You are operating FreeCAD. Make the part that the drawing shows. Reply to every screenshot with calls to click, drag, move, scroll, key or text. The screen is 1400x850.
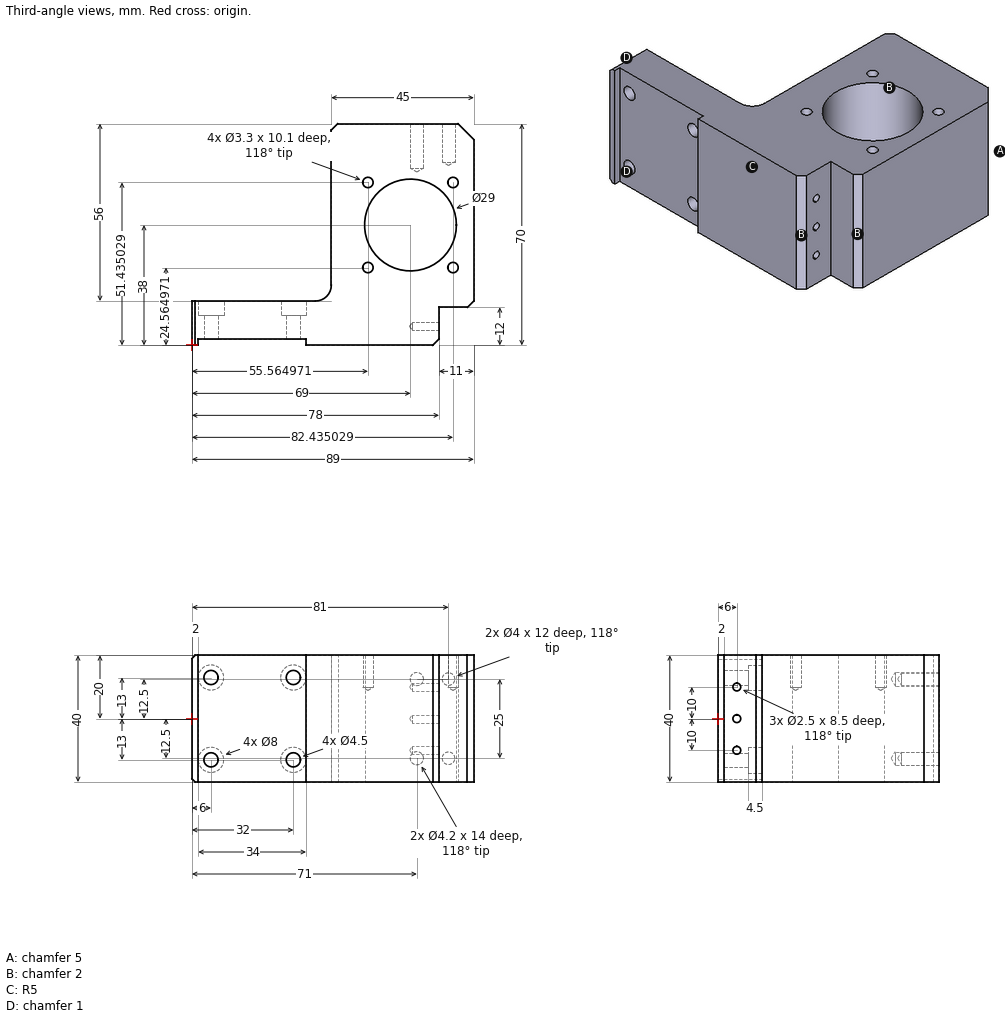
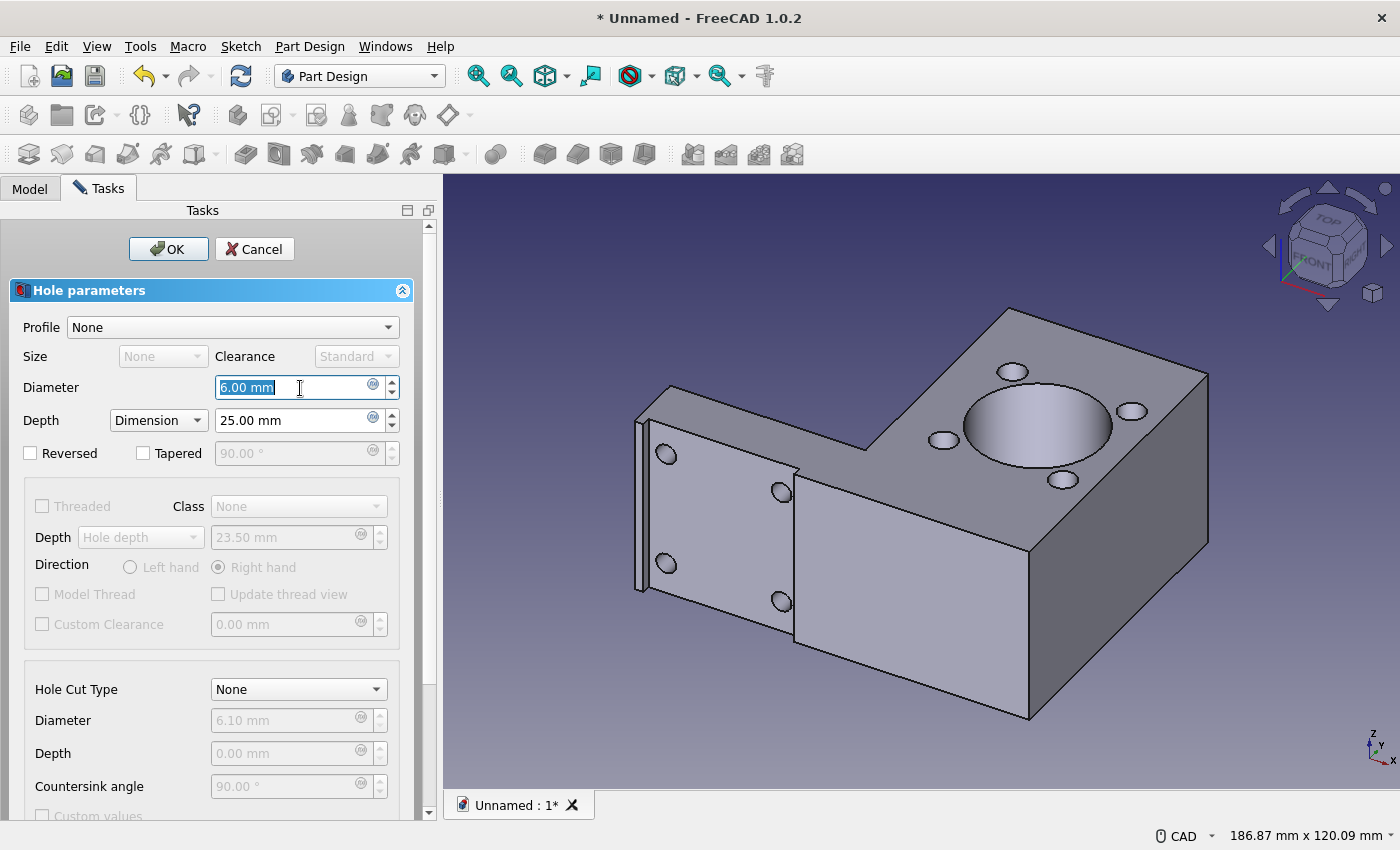
text(3.3)
key(Tab)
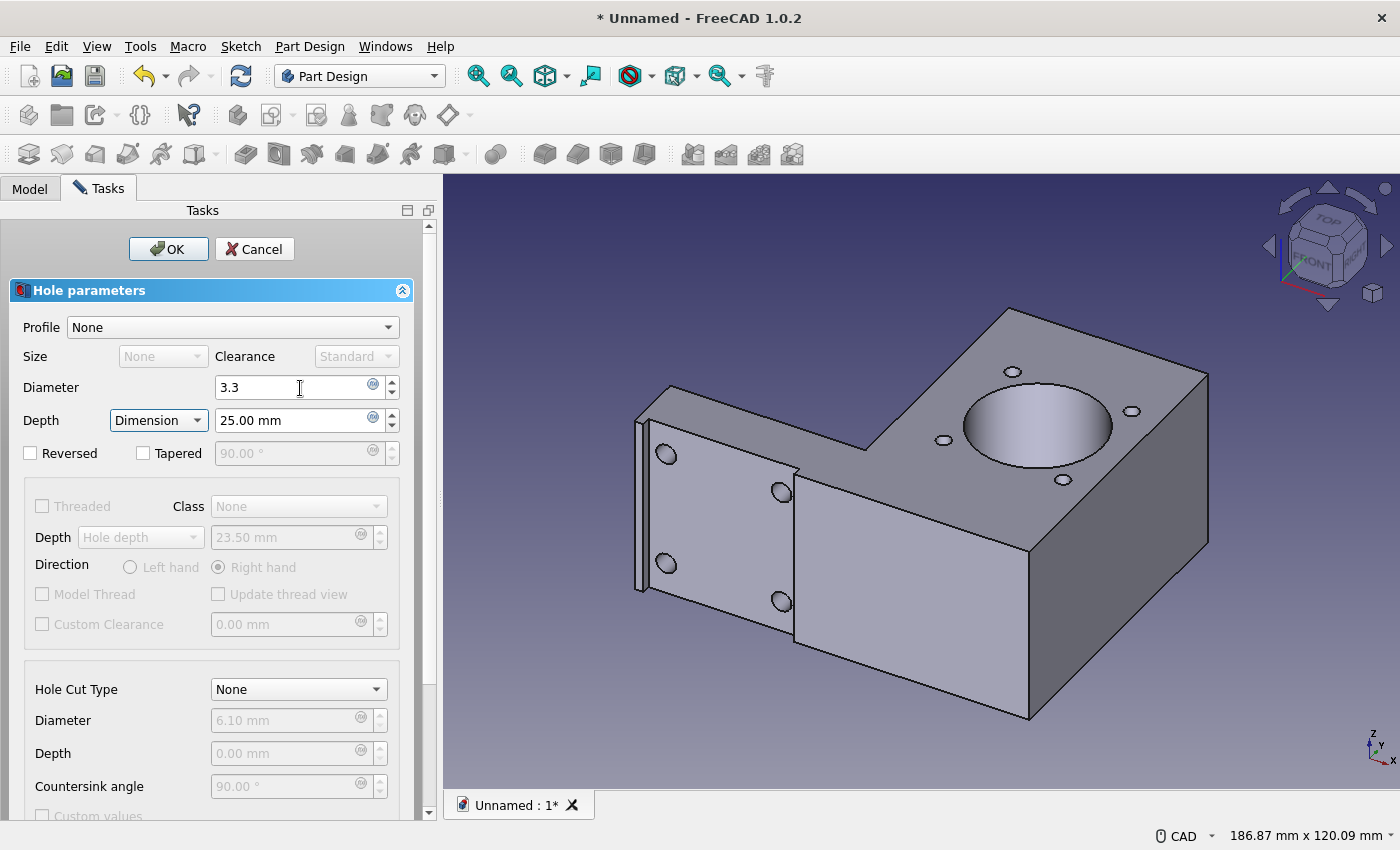
triple_click(300, 420)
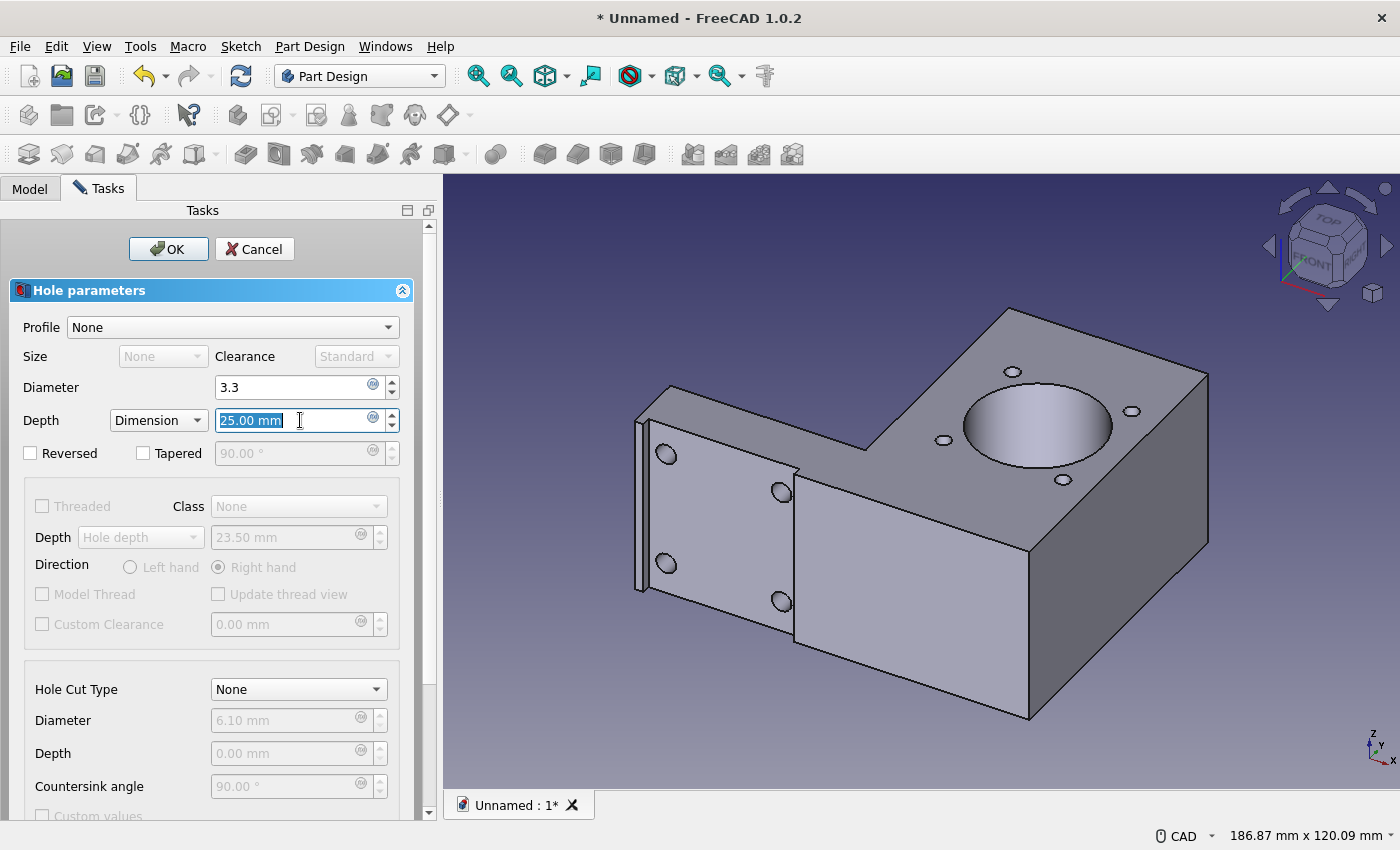
text(10.1)
key(Tab)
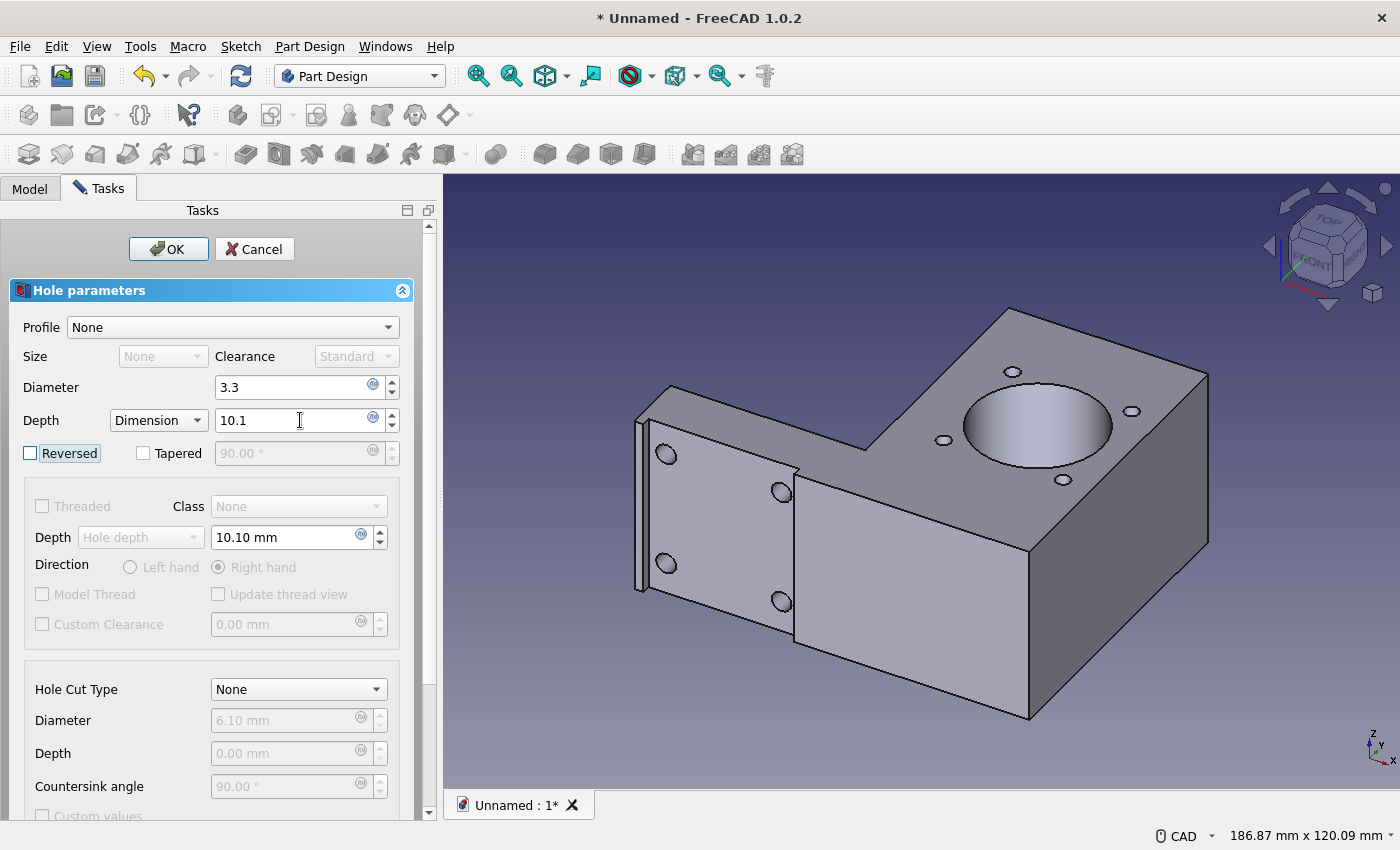
click(169, 249)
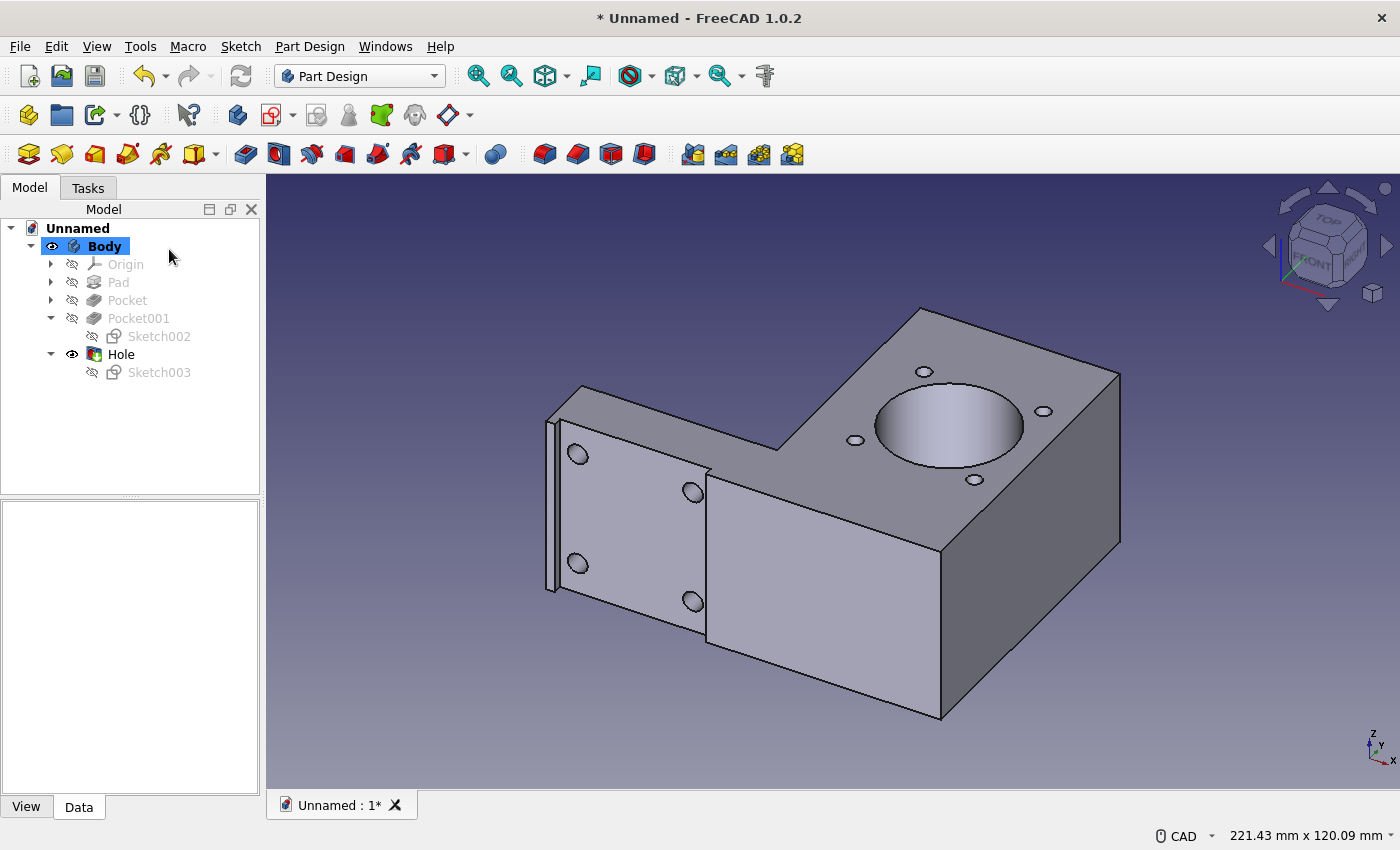
key(4)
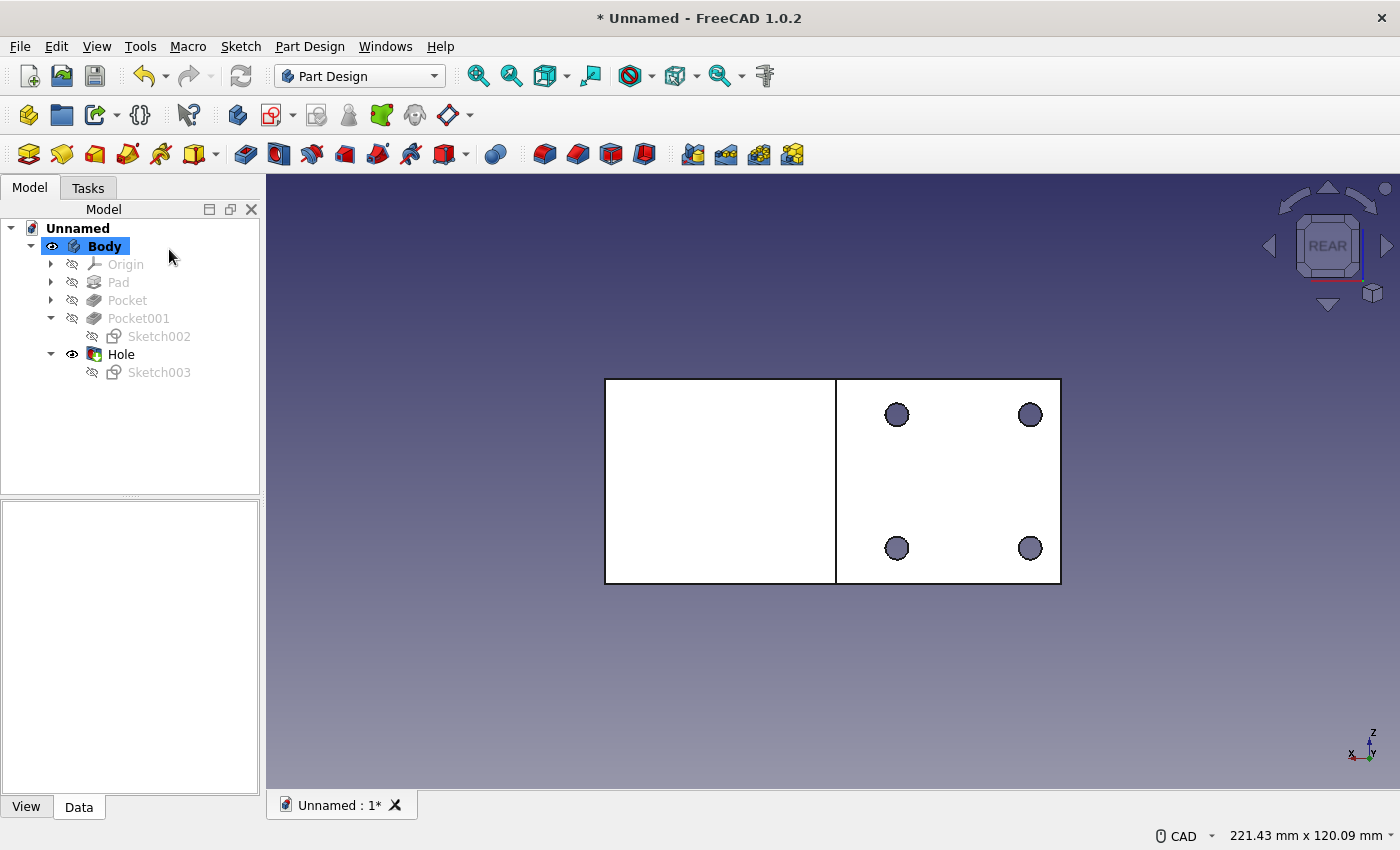
click(479, 76)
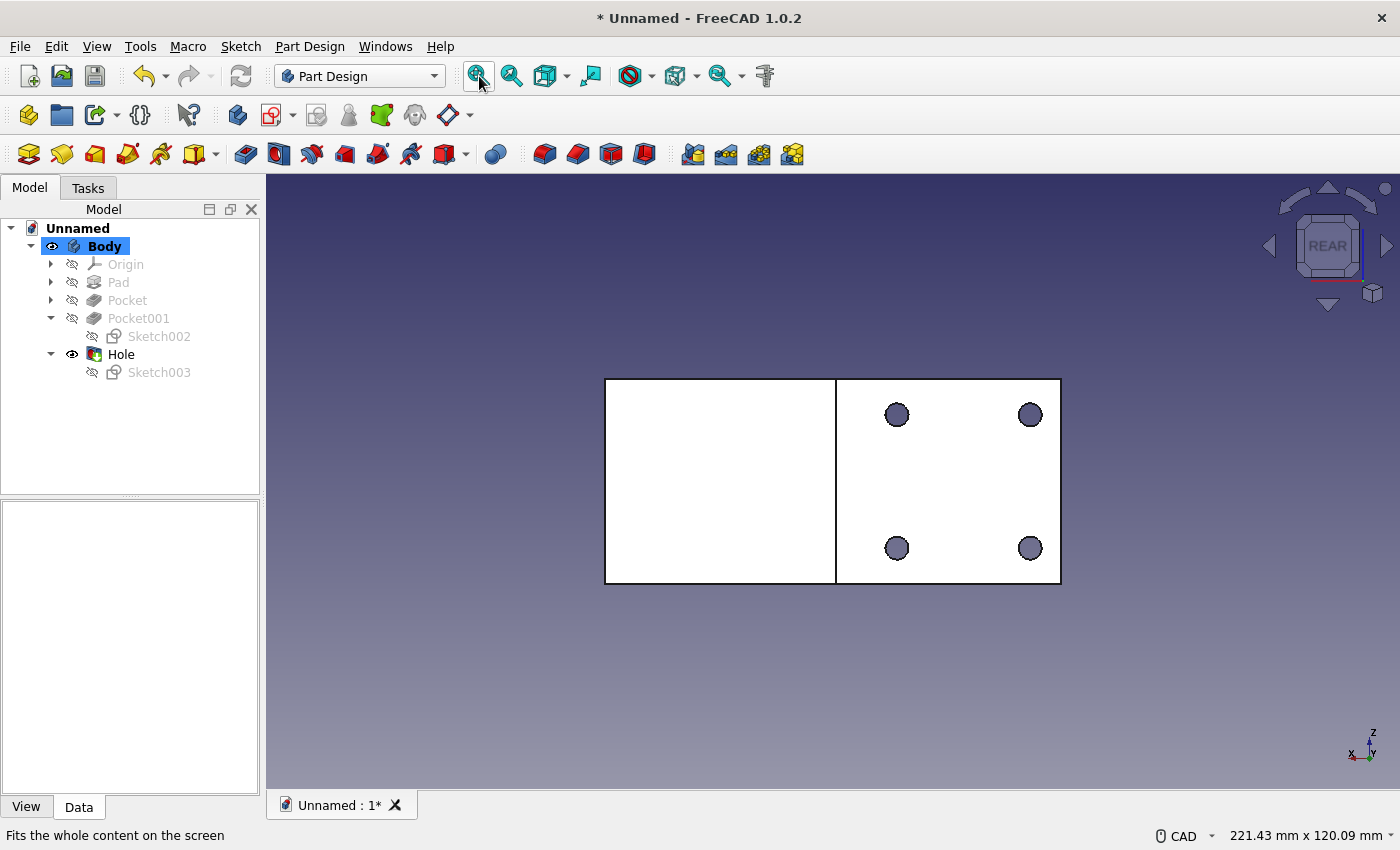
click(720, 481)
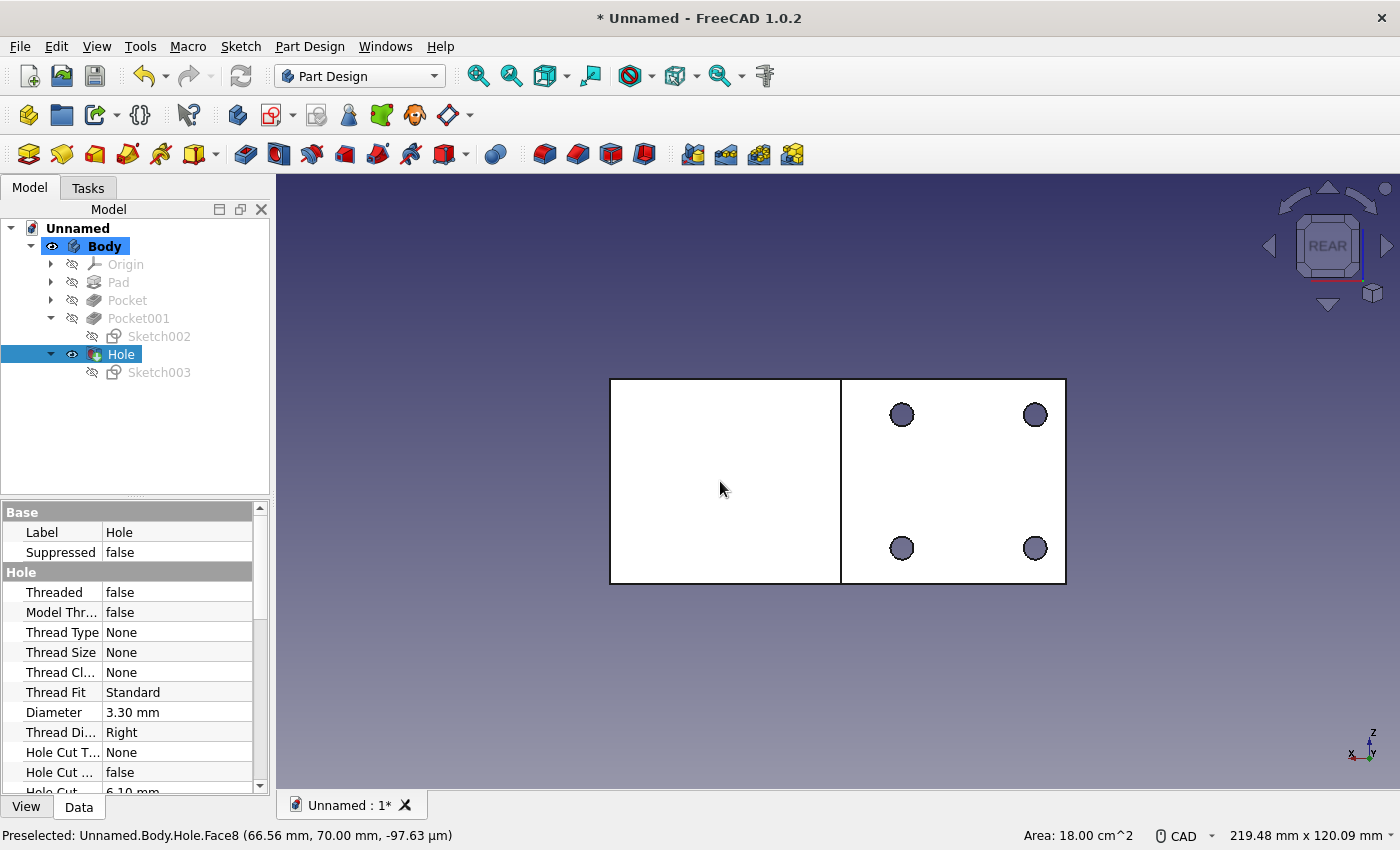
click(270, 116)